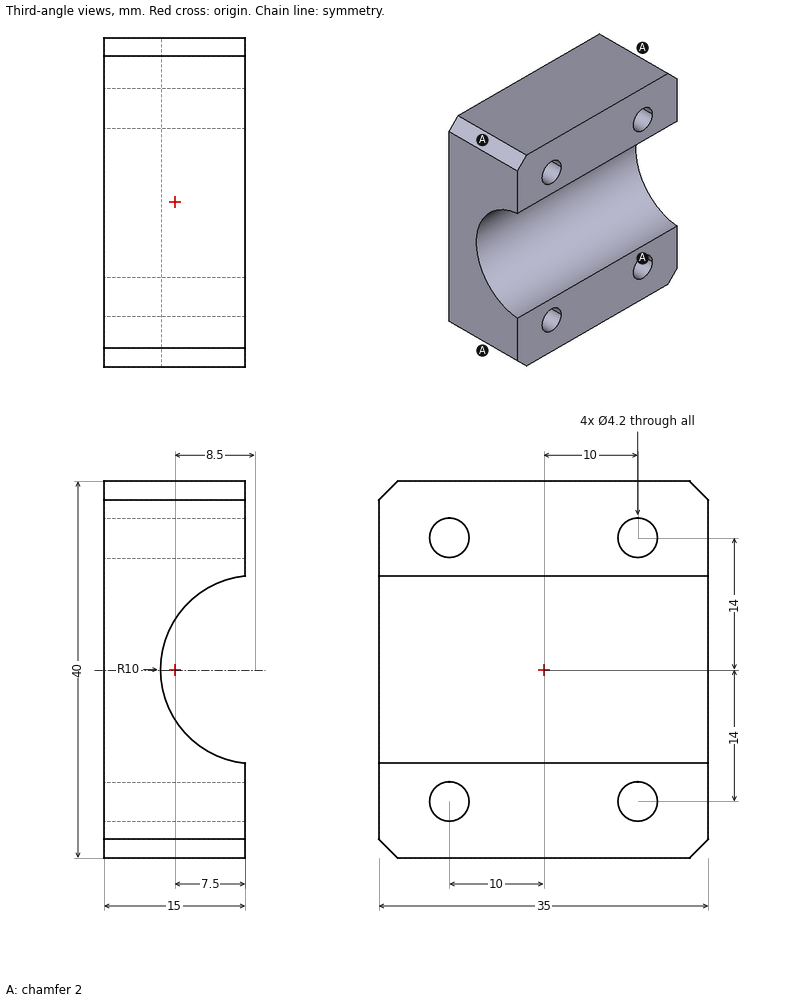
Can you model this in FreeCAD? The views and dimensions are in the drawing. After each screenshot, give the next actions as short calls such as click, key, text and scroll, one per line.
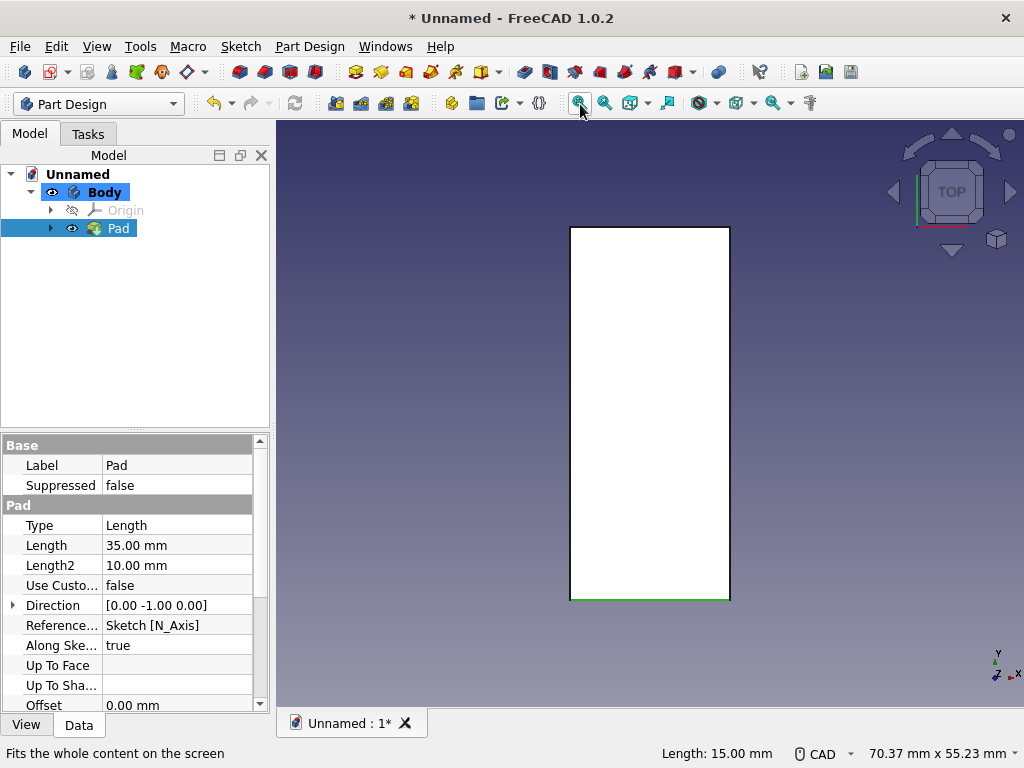
click(650, 226, ctrl)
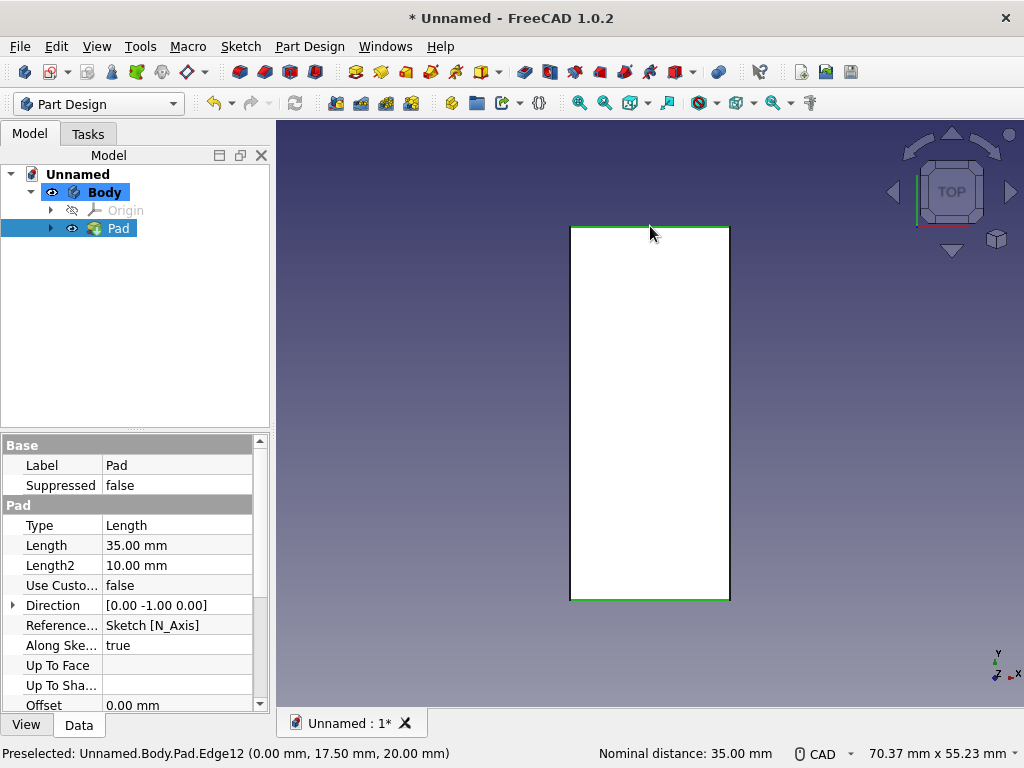
key(1)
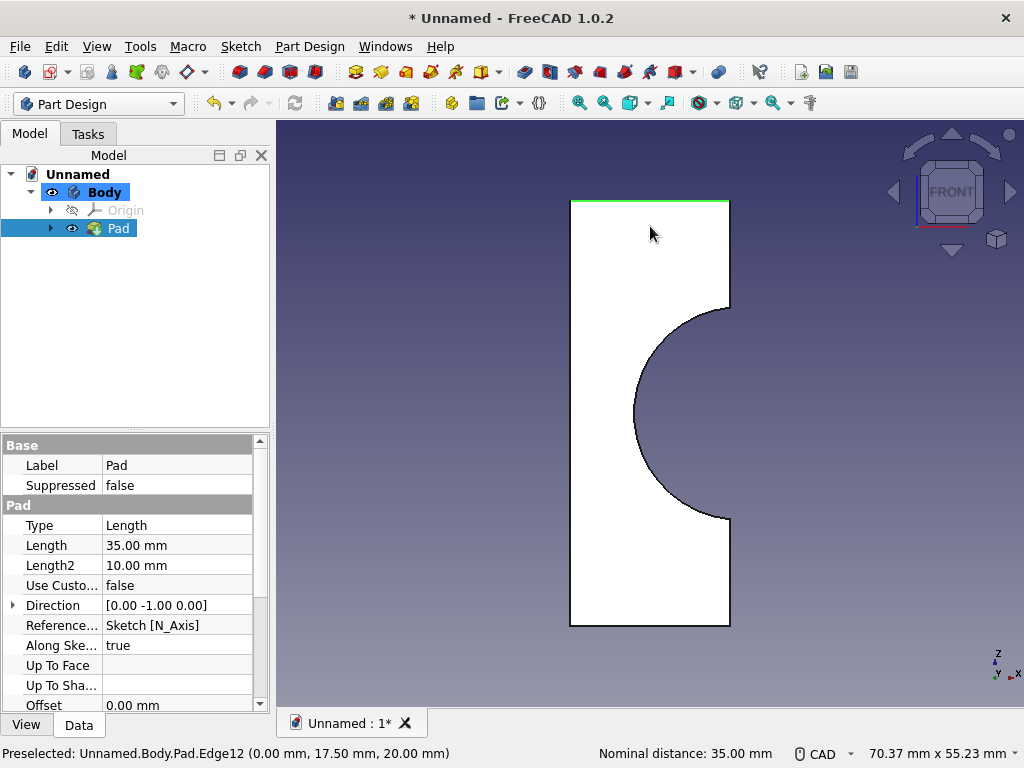
key(3)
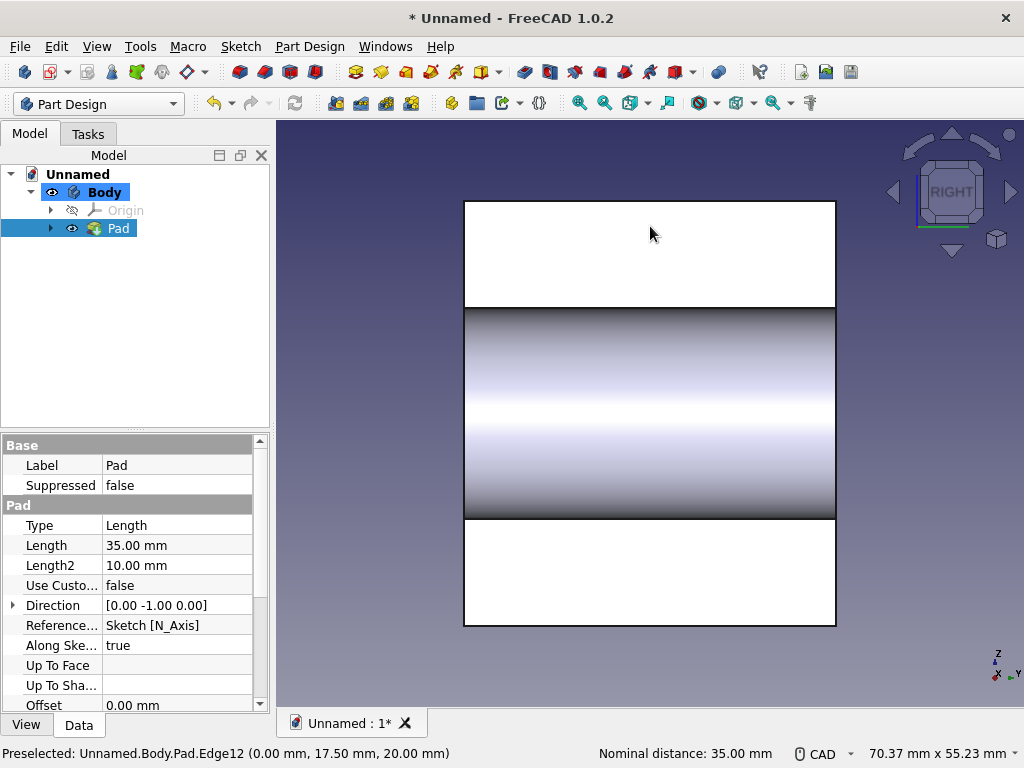
key(5)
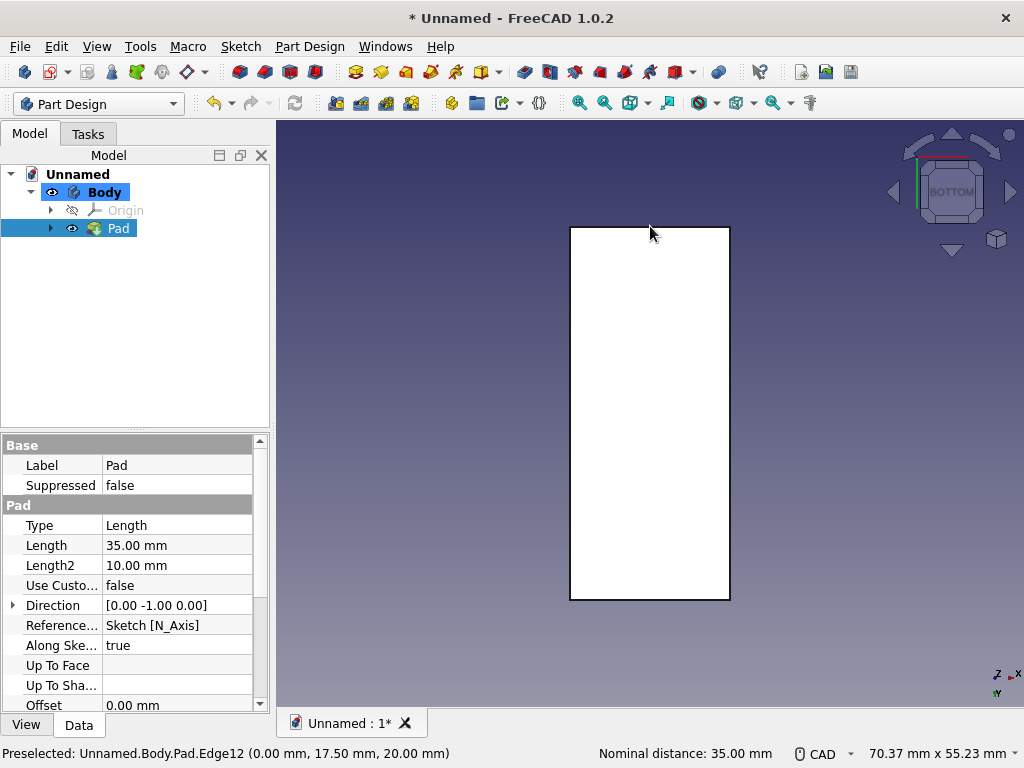
click(650, 226, ctrl)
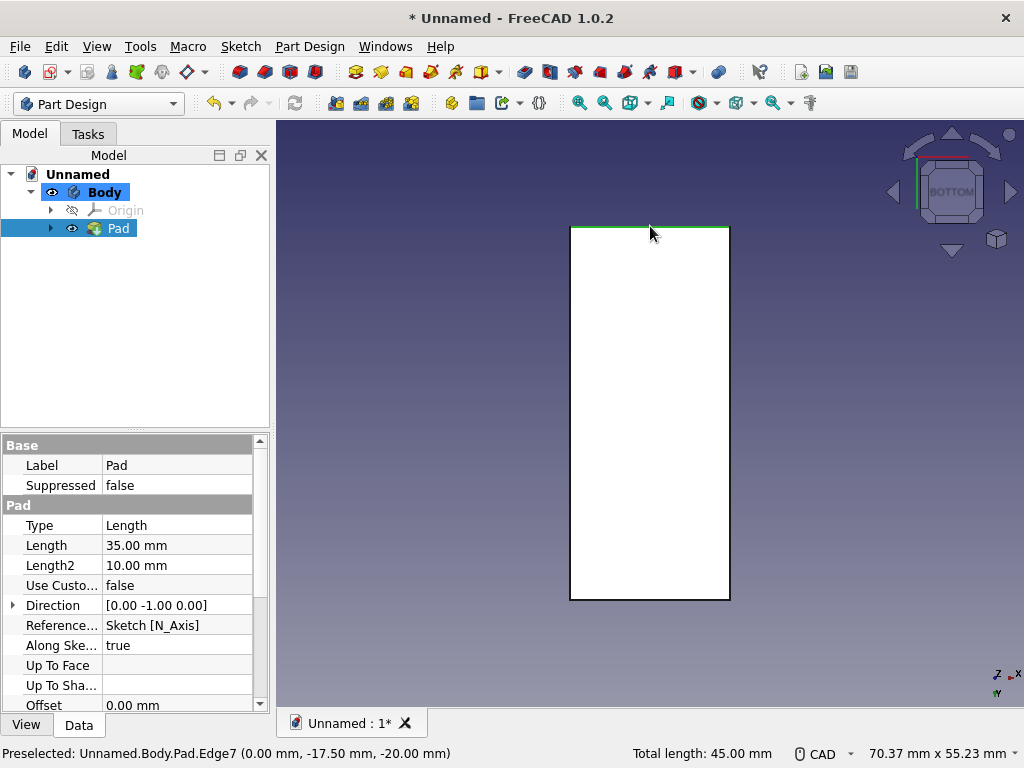
key(4)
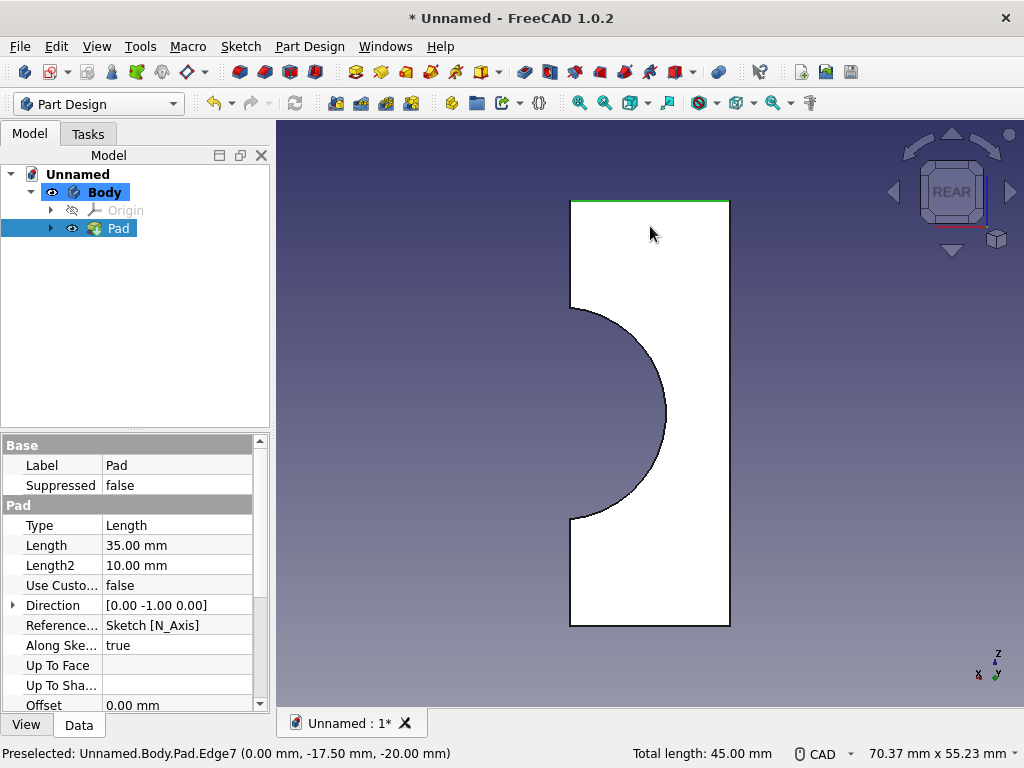
click(650, 625, ctrl)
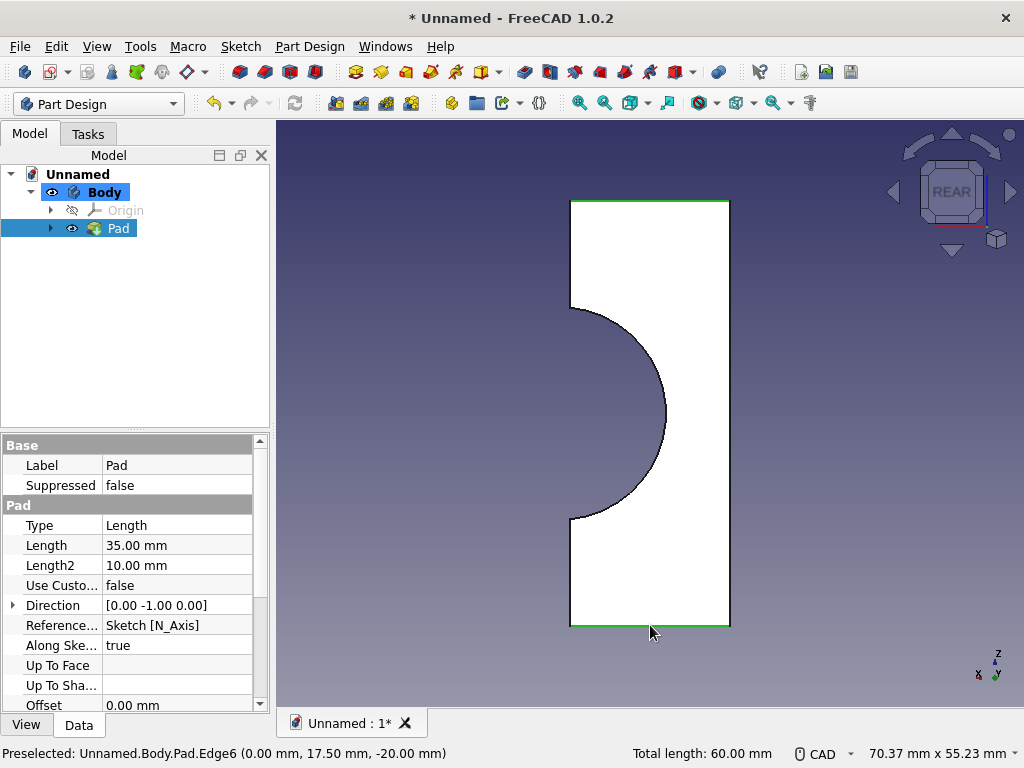
click(265, 72)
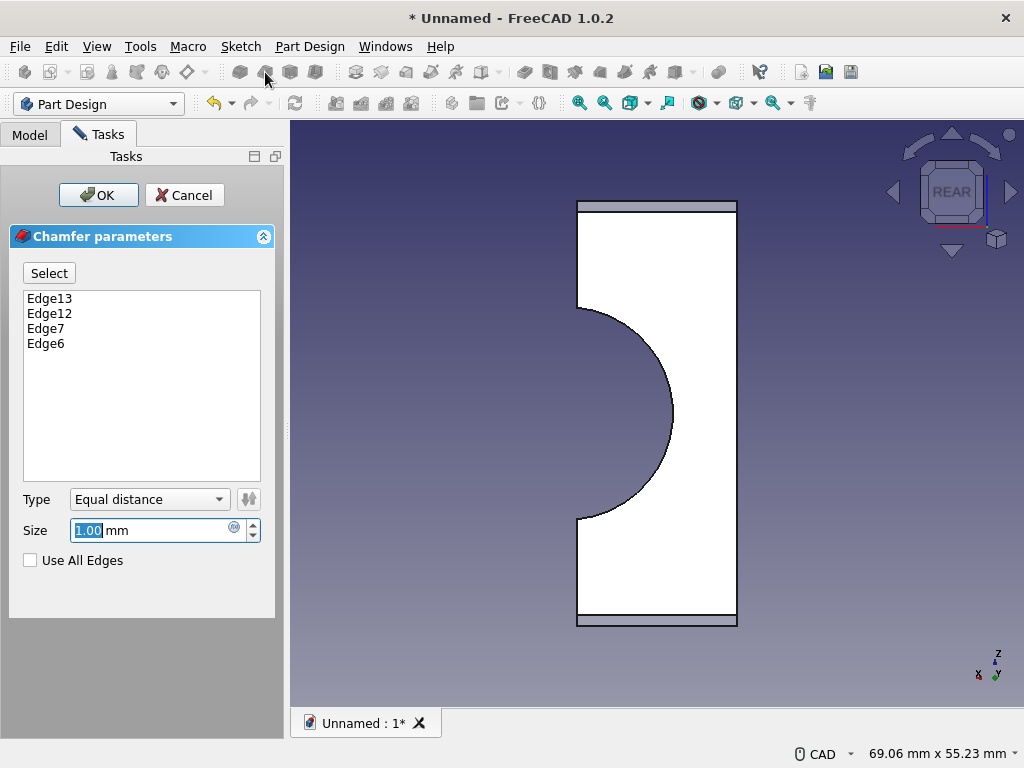
text(2)
key(Tab)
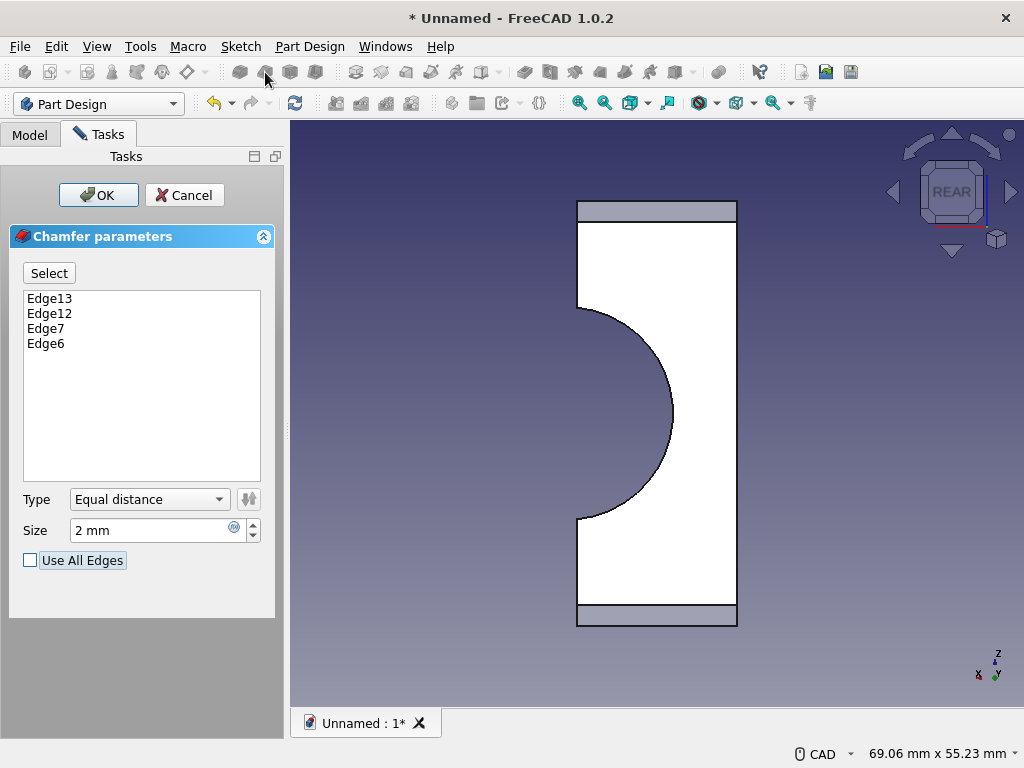
click(99, 195)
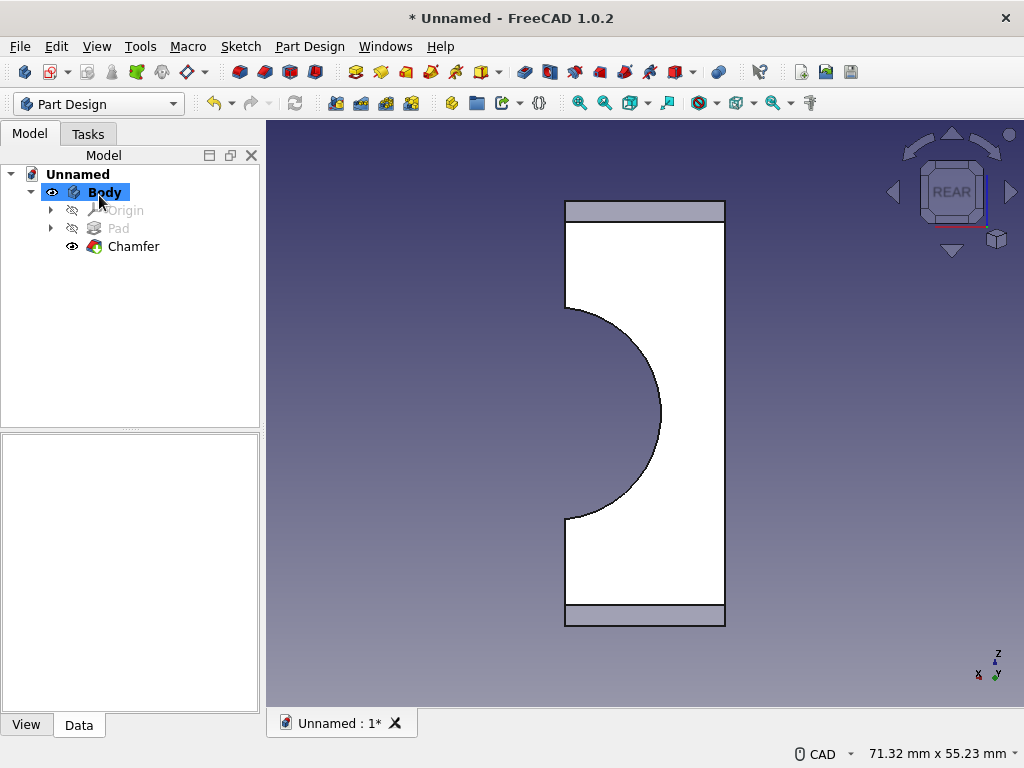
key(0)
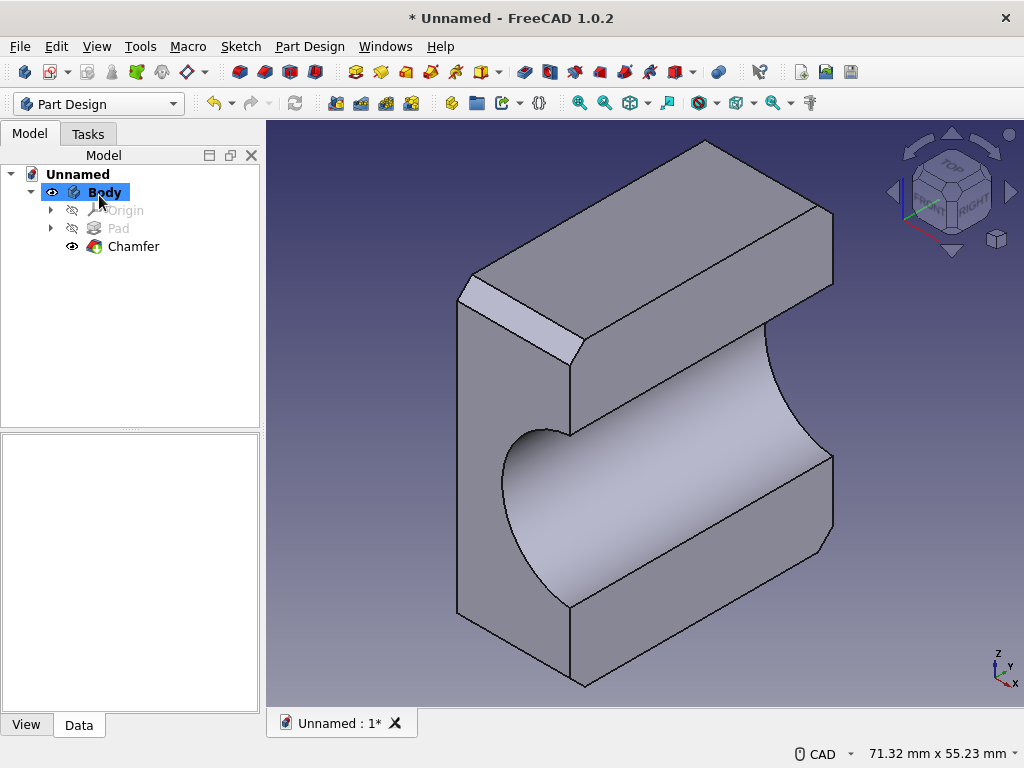
click(777, 532)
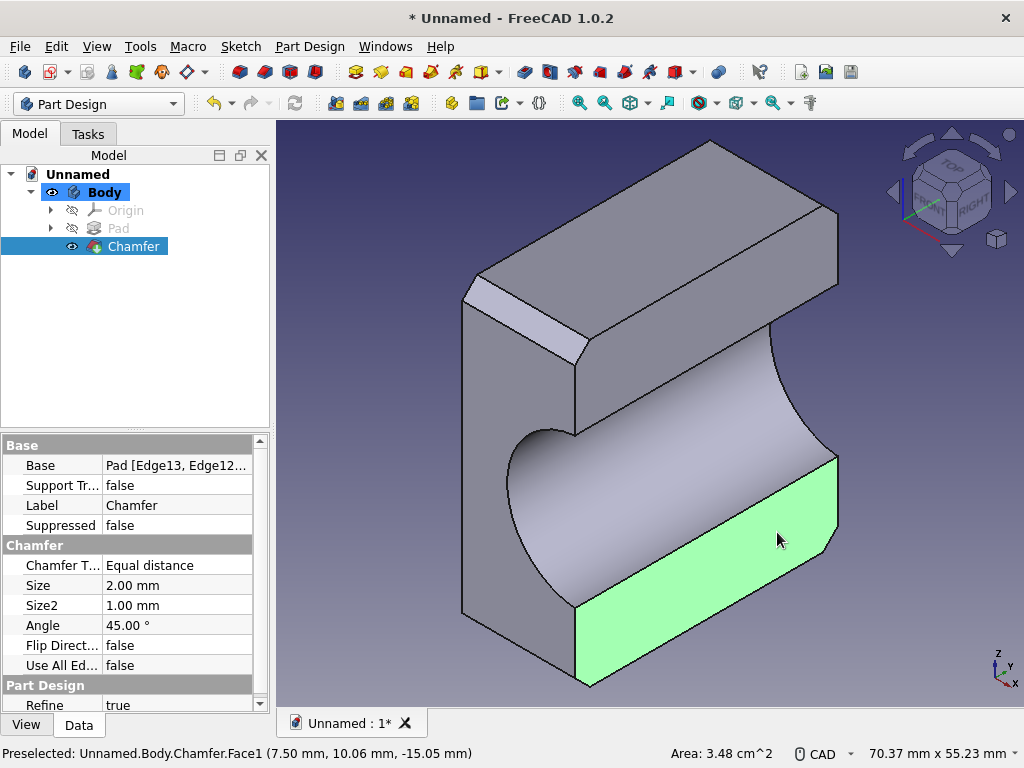
click(50, 72)